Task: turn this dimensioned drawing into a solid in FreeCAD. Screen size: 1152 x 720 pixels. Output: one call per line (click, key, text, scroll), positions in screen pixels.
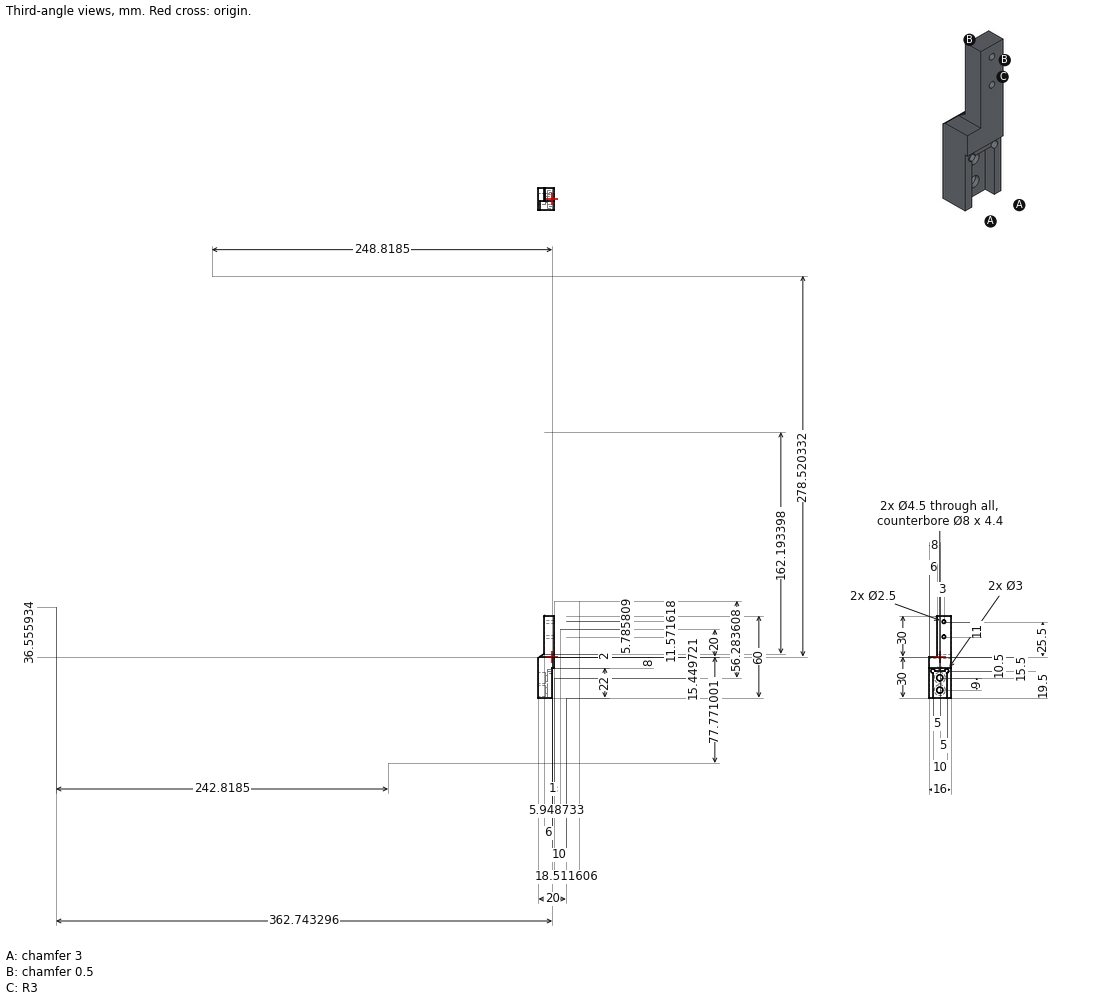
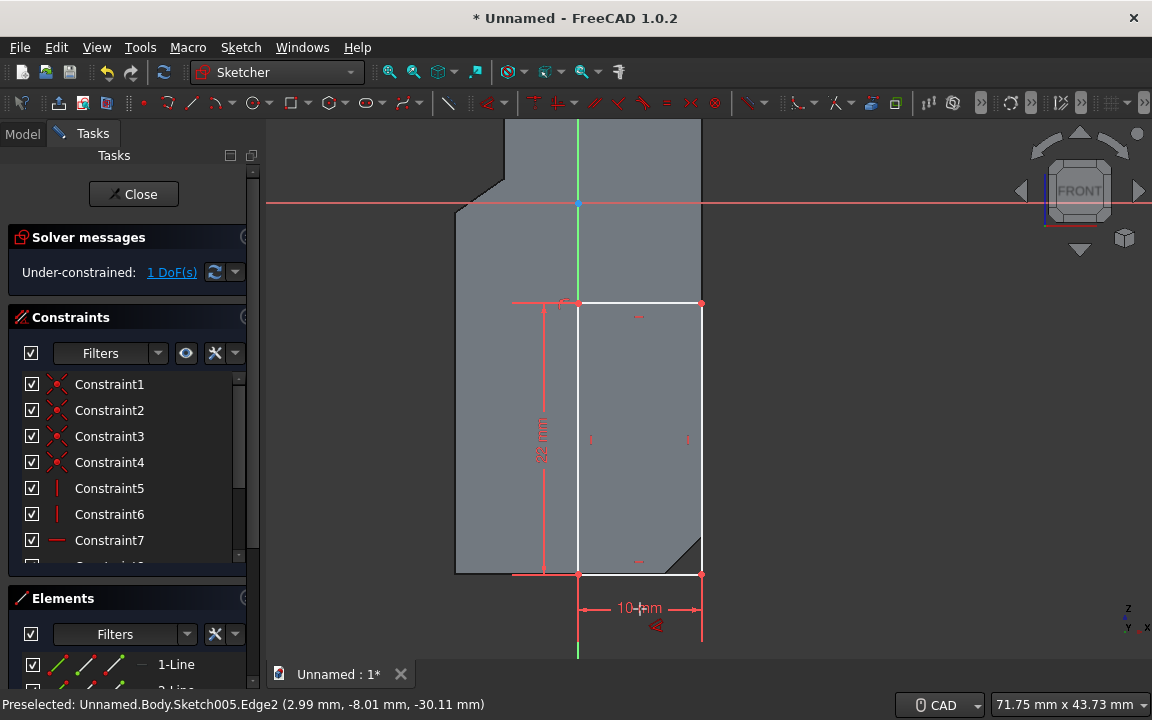
click(578, 303)
click(544, 253)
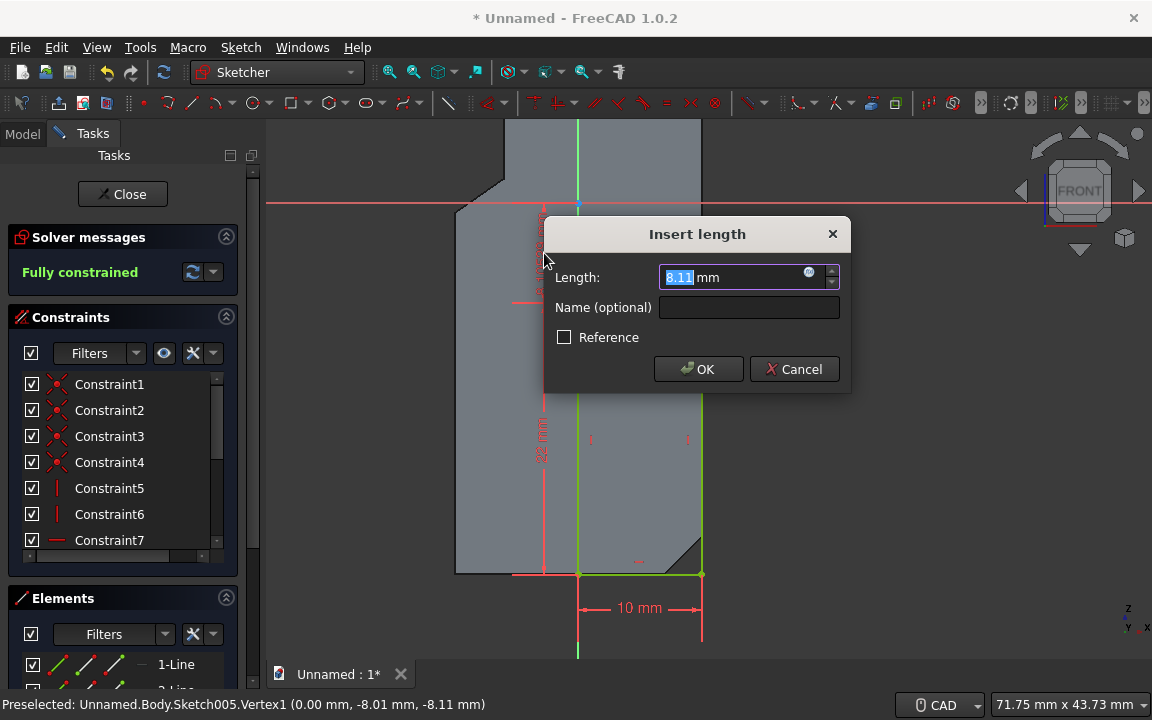
text(8)
key(Return)
key(Escape)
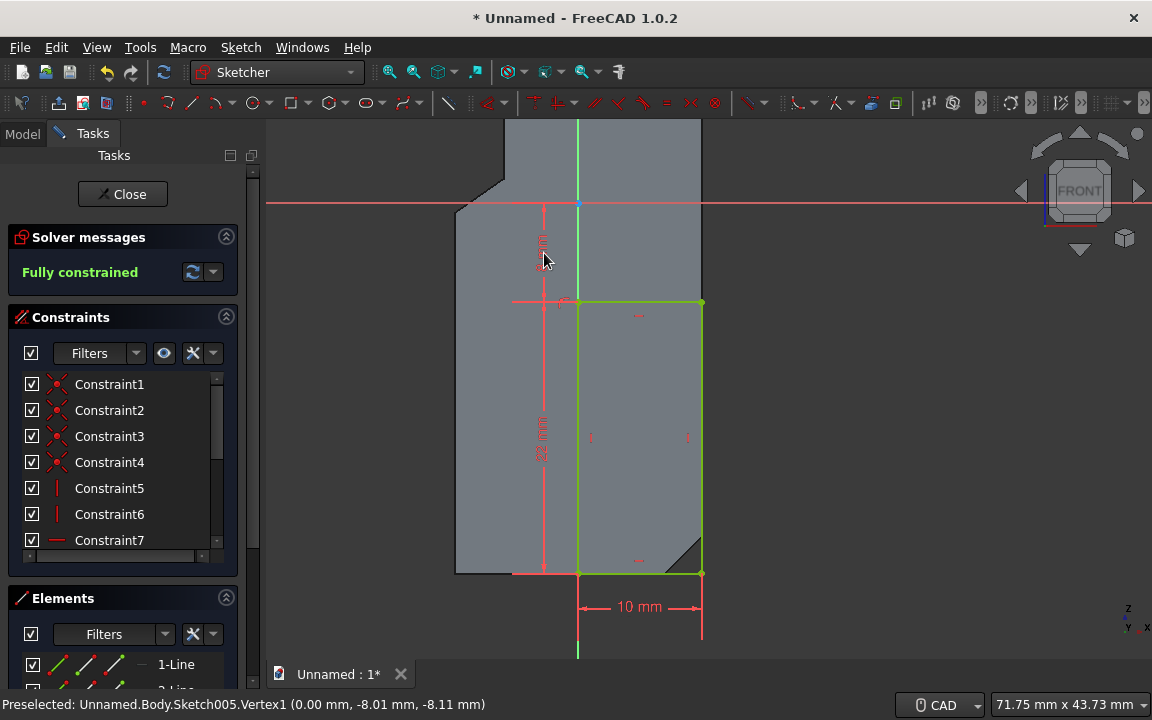
click(123, 194)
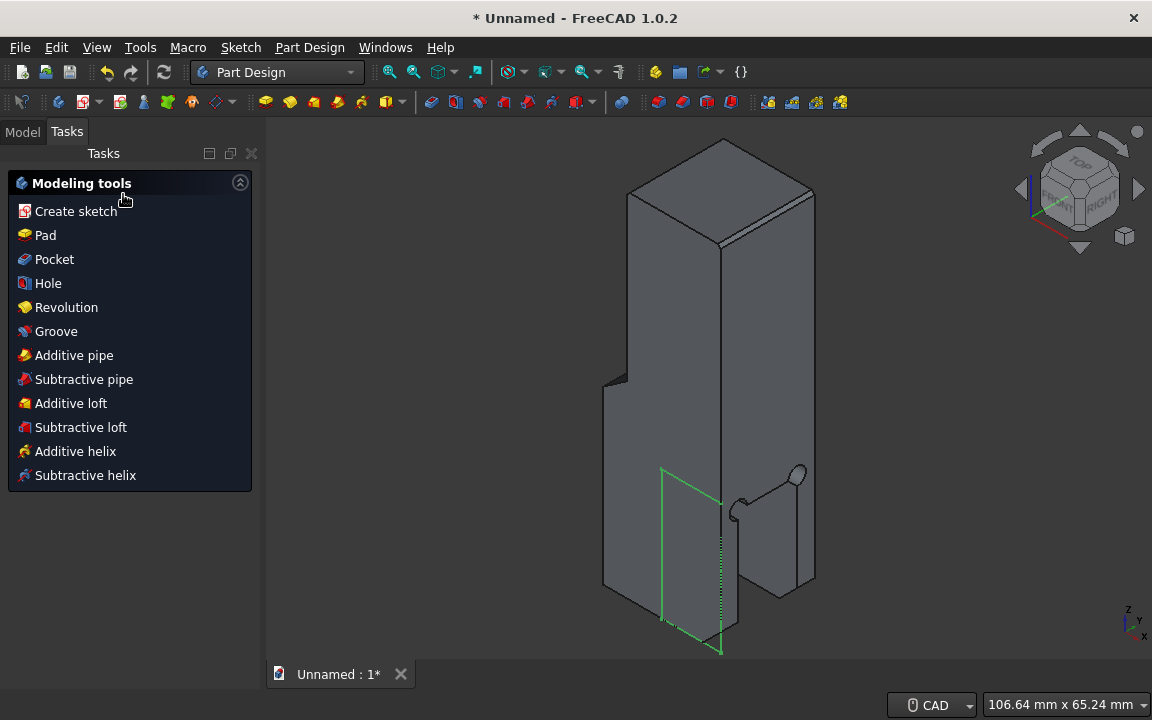
click(432, 102)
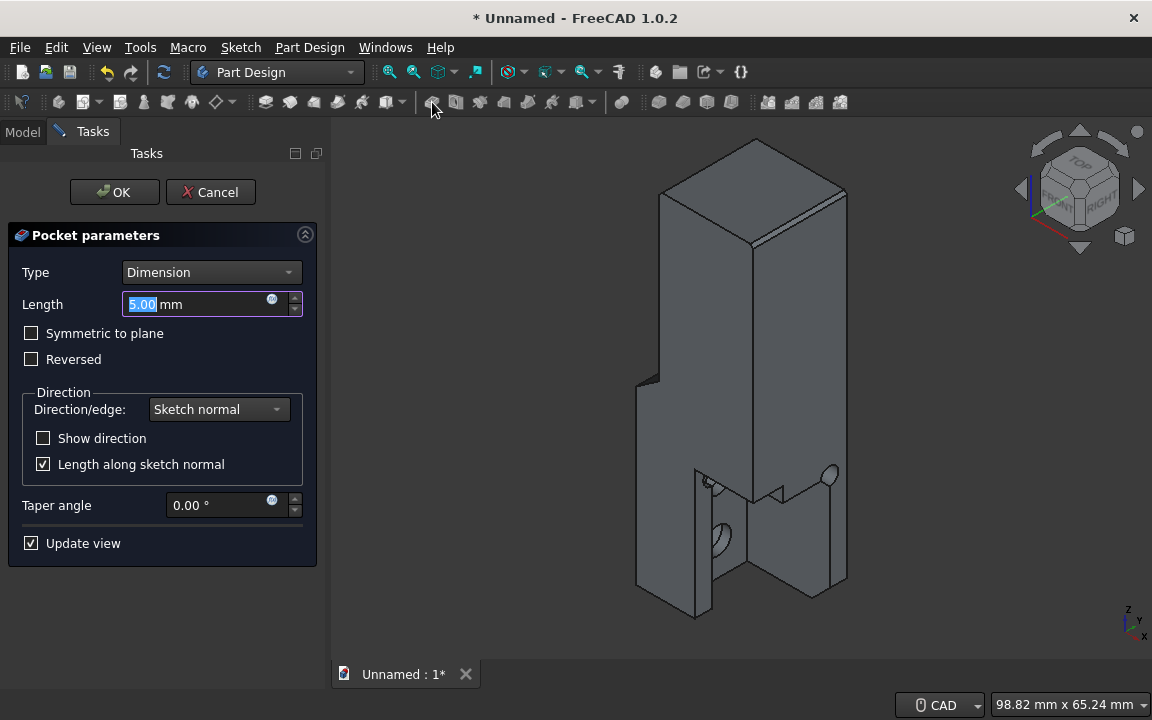
click(212, 272)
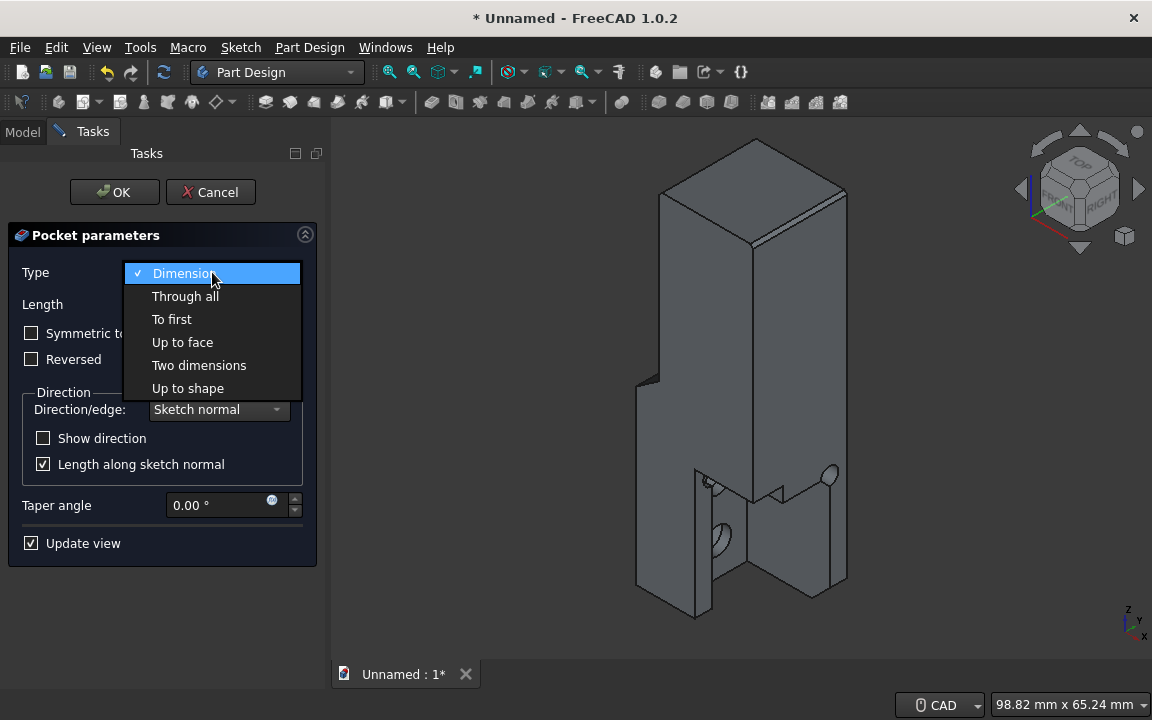
click(212, 296)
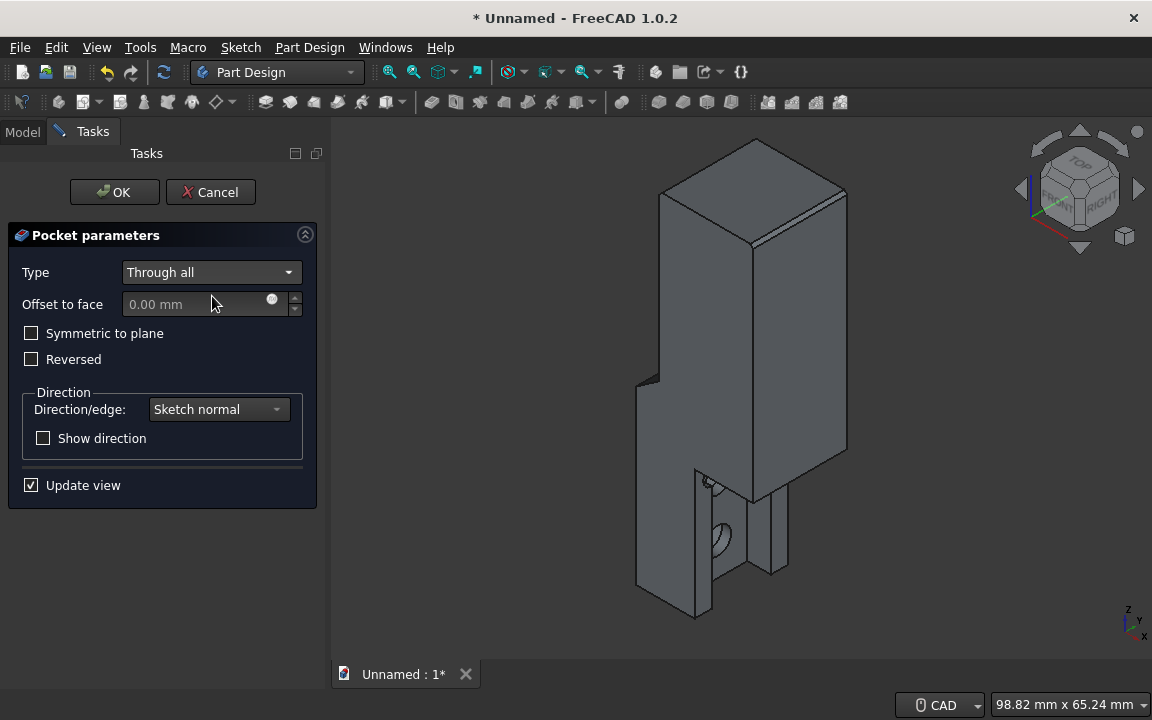
click(115, 192)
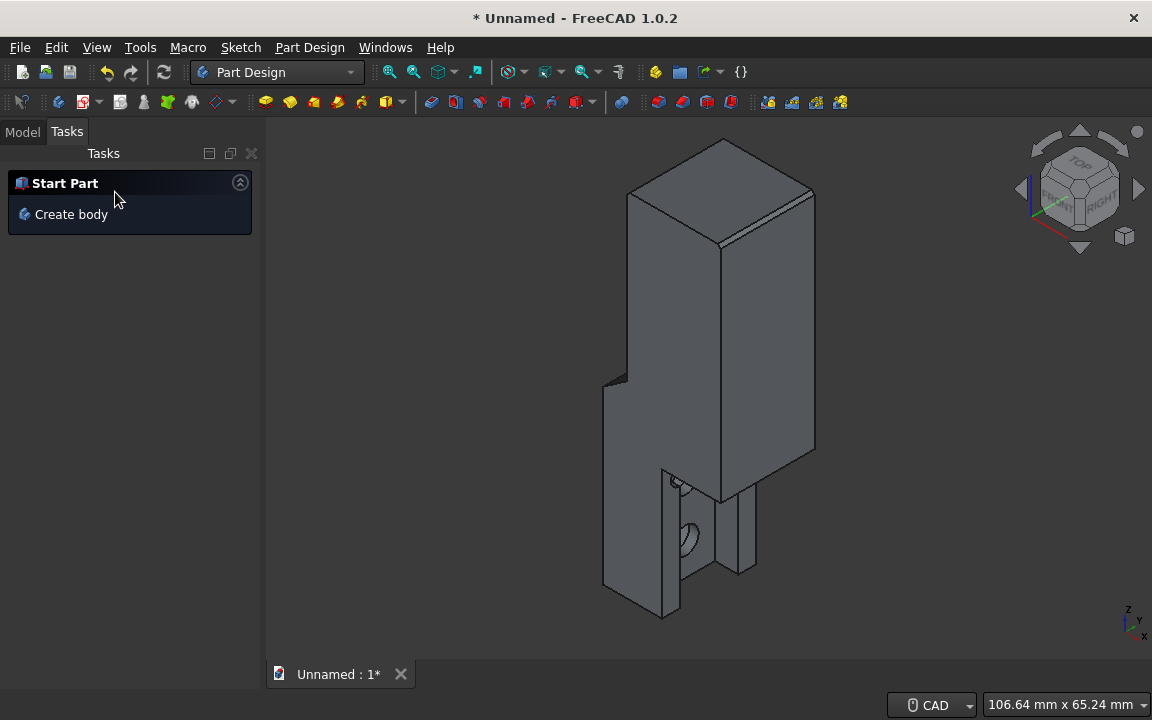
click(768, 312)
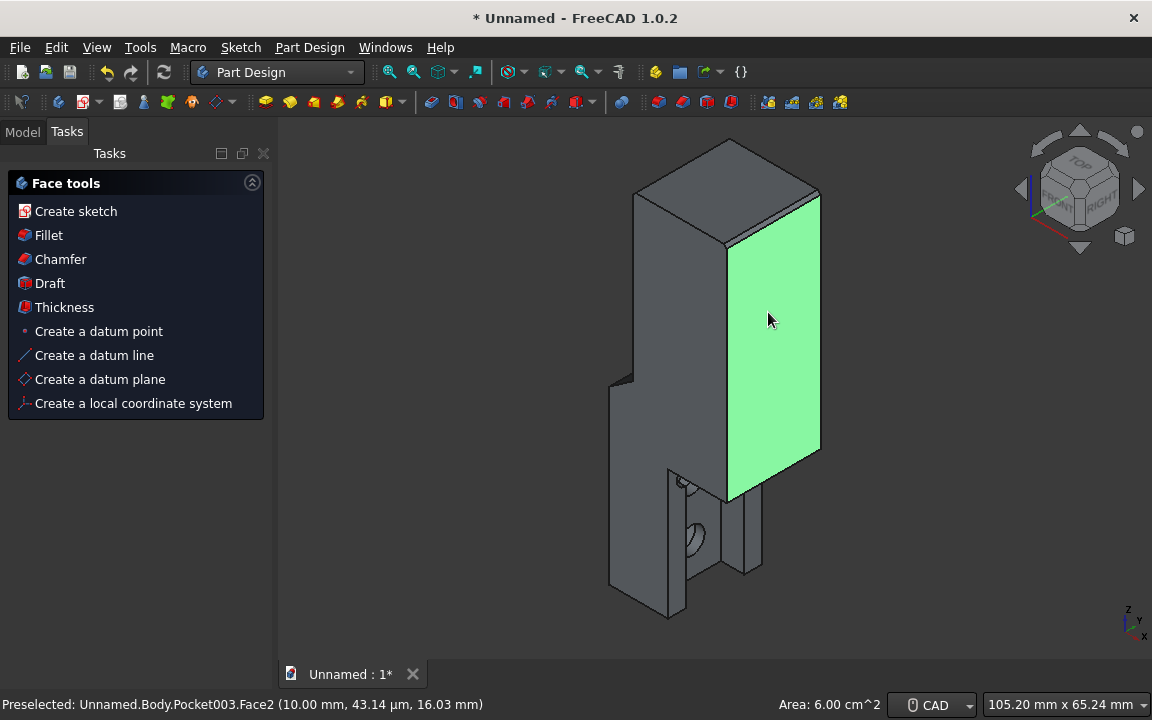
click(84, 102)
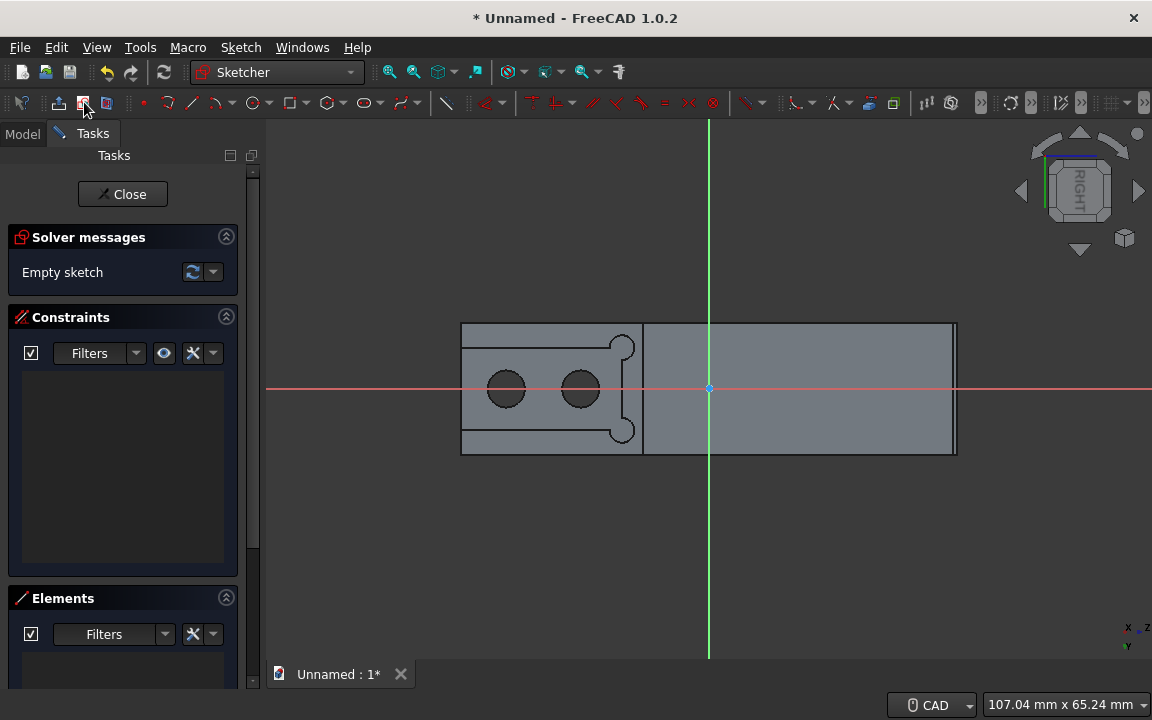
scroll(987, 316, up, 3)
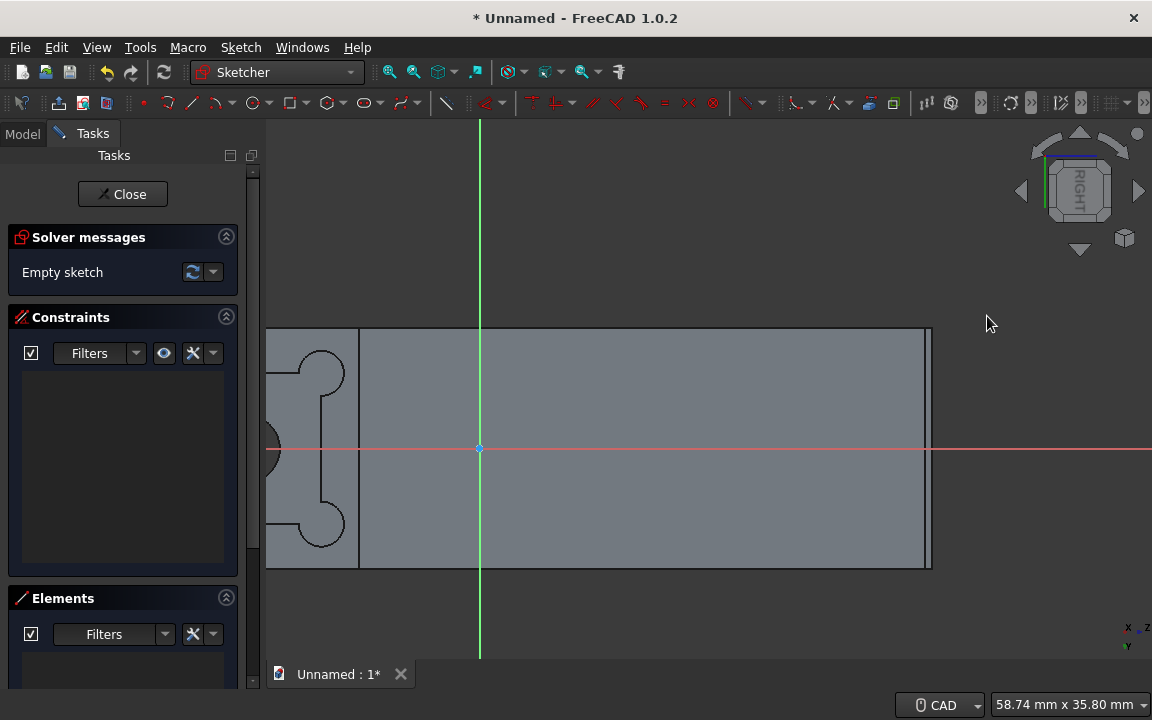
key(g)
key(r)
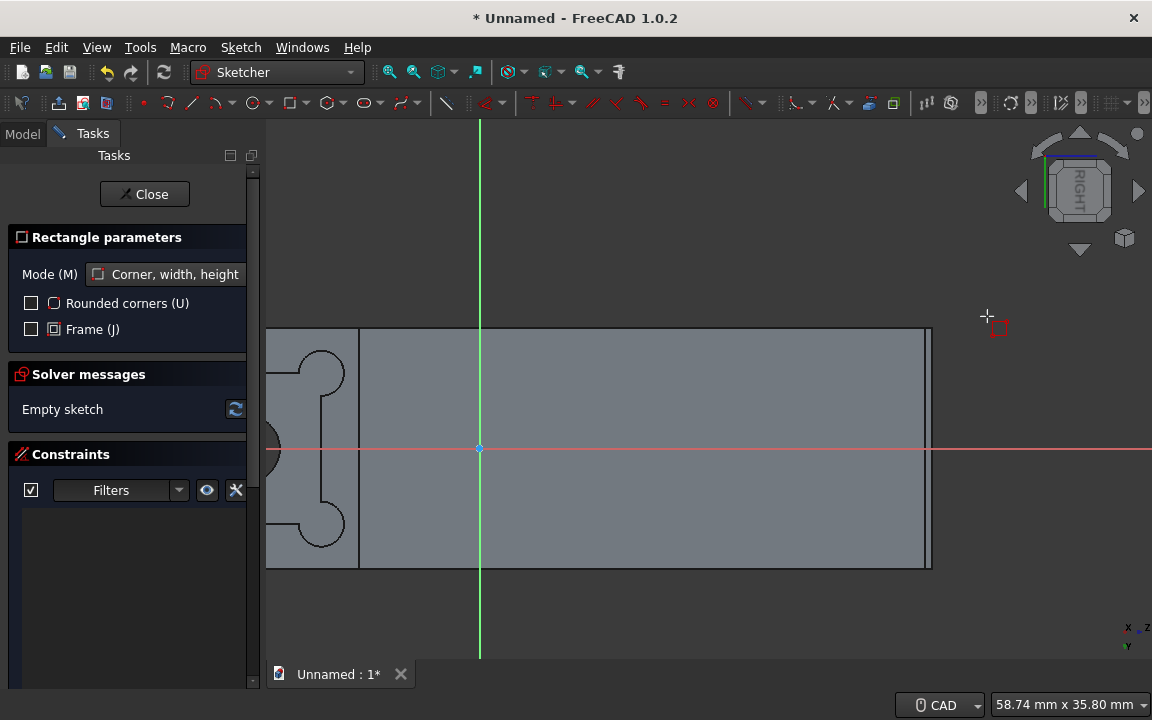
click(480, 328)
click(932, 419)
key(Escape)